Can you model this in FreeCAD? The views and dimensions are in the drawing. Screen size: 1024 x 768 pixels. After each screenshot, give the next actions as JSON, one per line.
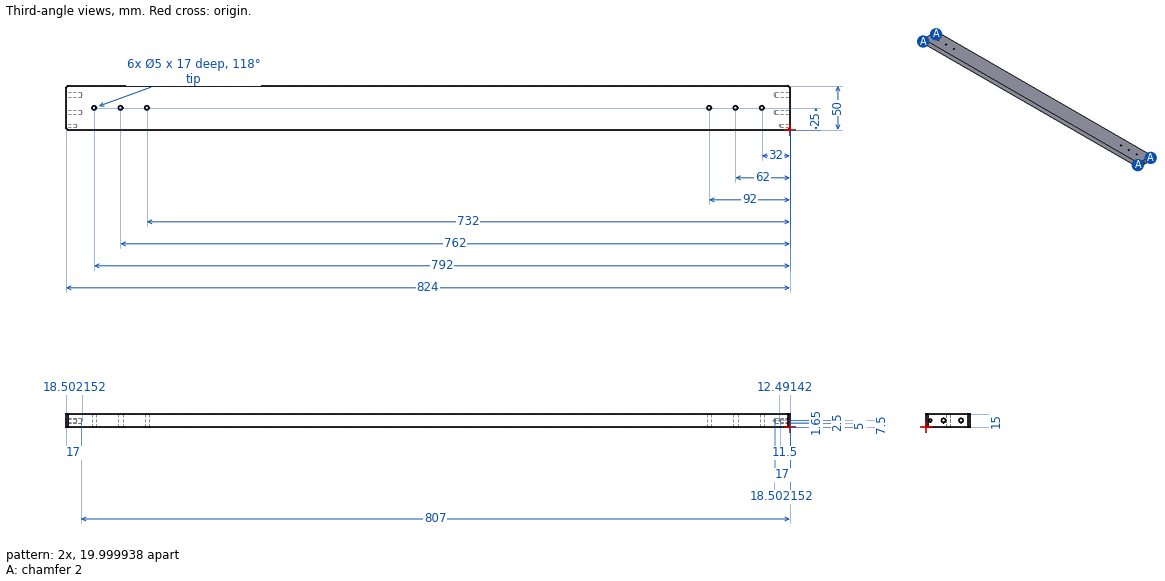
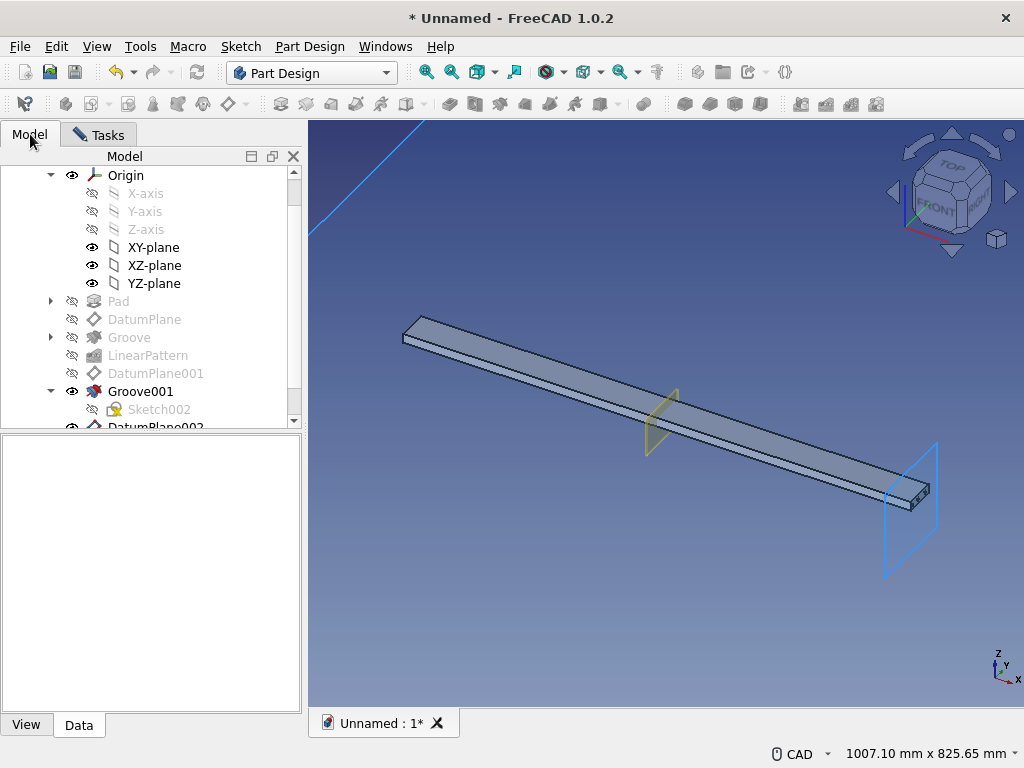
{"action": "left_click", "coordinate": [117, 427]}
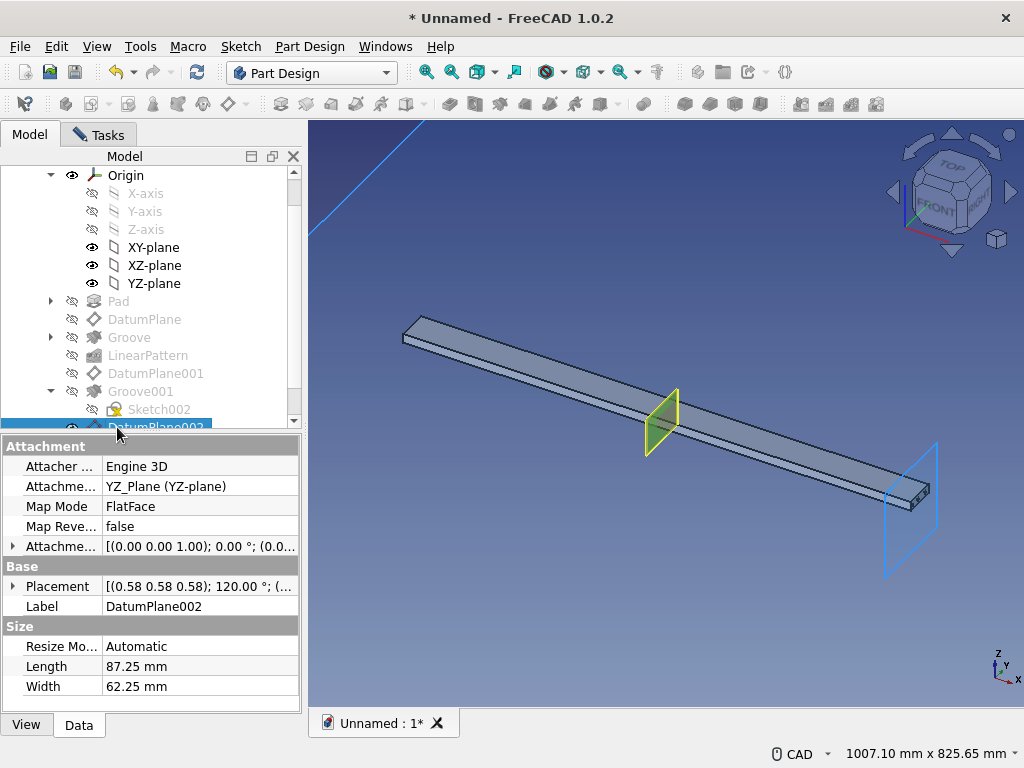
{"action": "left_click", "coordinate": [98, 134]}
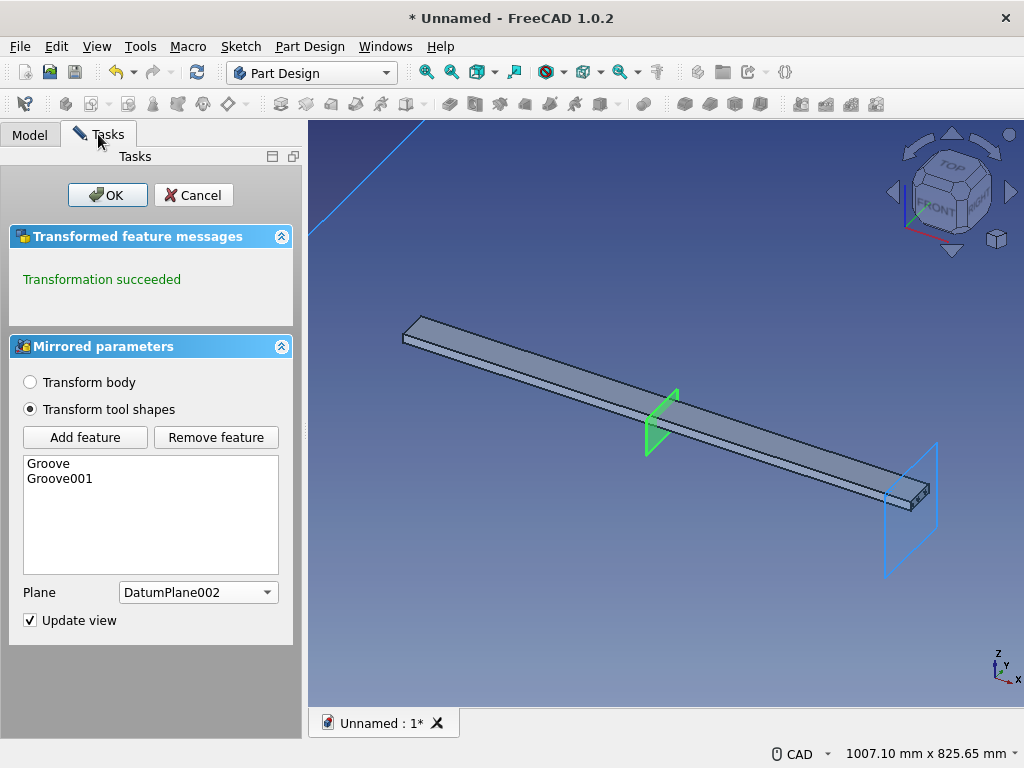
{"action": "left_click", "coordinate": [108, 195]}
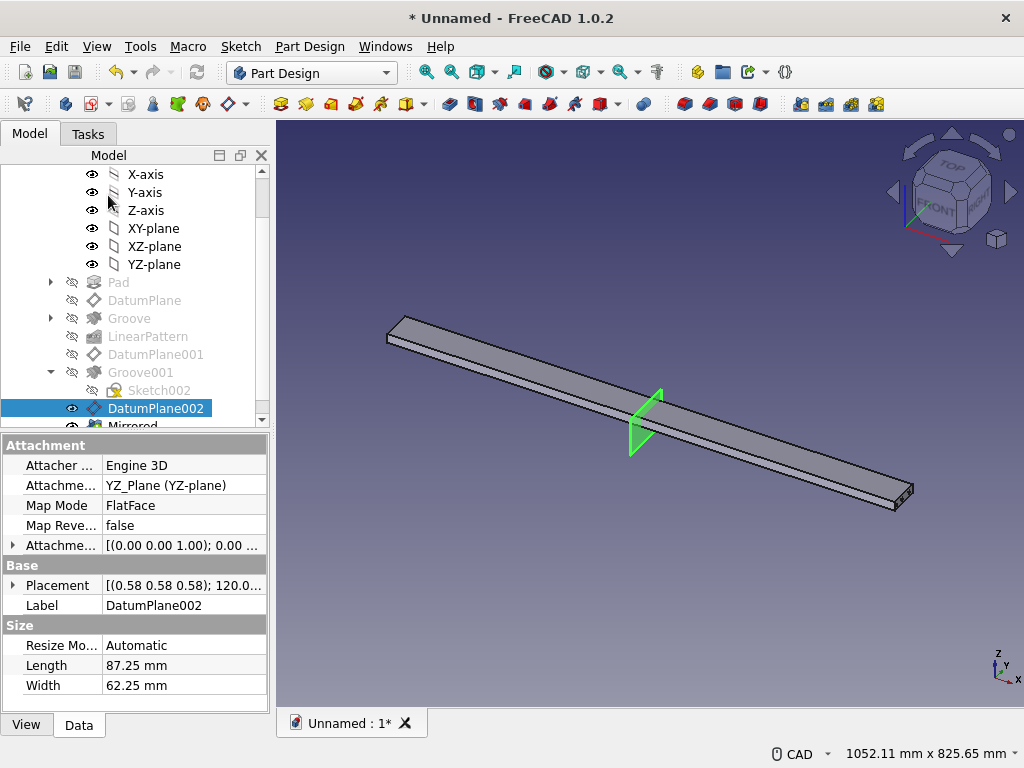
{"action": "left_click", "coordinate": [117, 408]}
{"action": "key", "text": "space"}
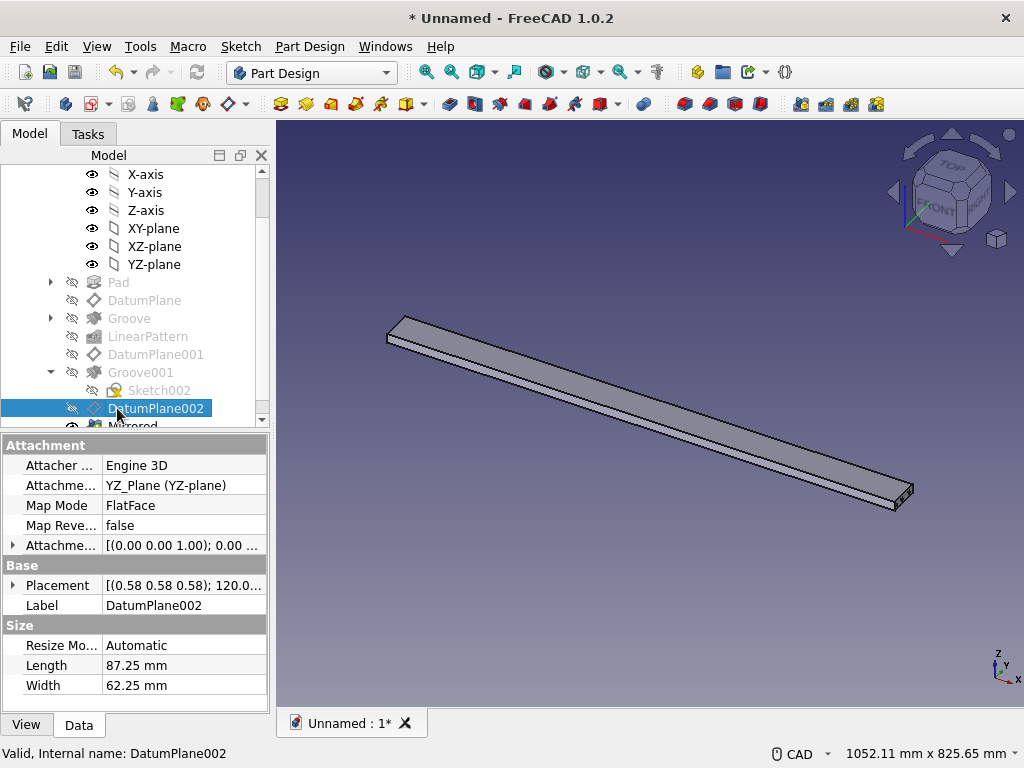
{"action": "scroll", "coordinate": [161, 296], "scroll_direction": "down", "scroll_amount": 3}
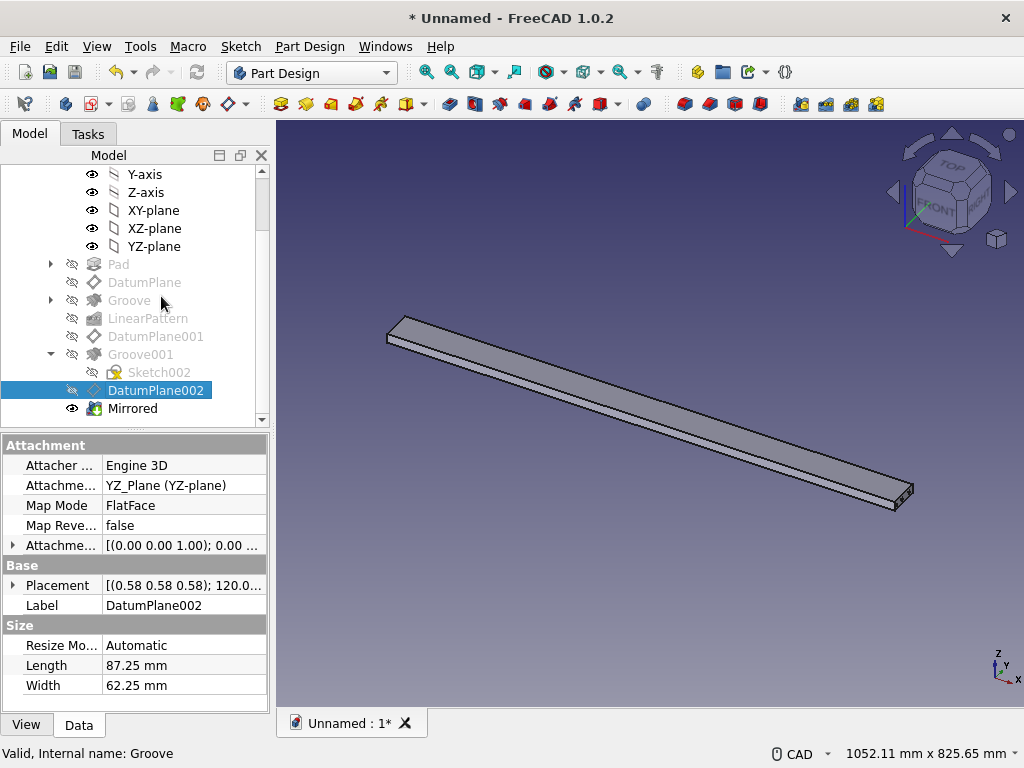
{"action": "scroll", "coordinate": [161, 296], "scroll_direction": "up", "scroll_amount": 15}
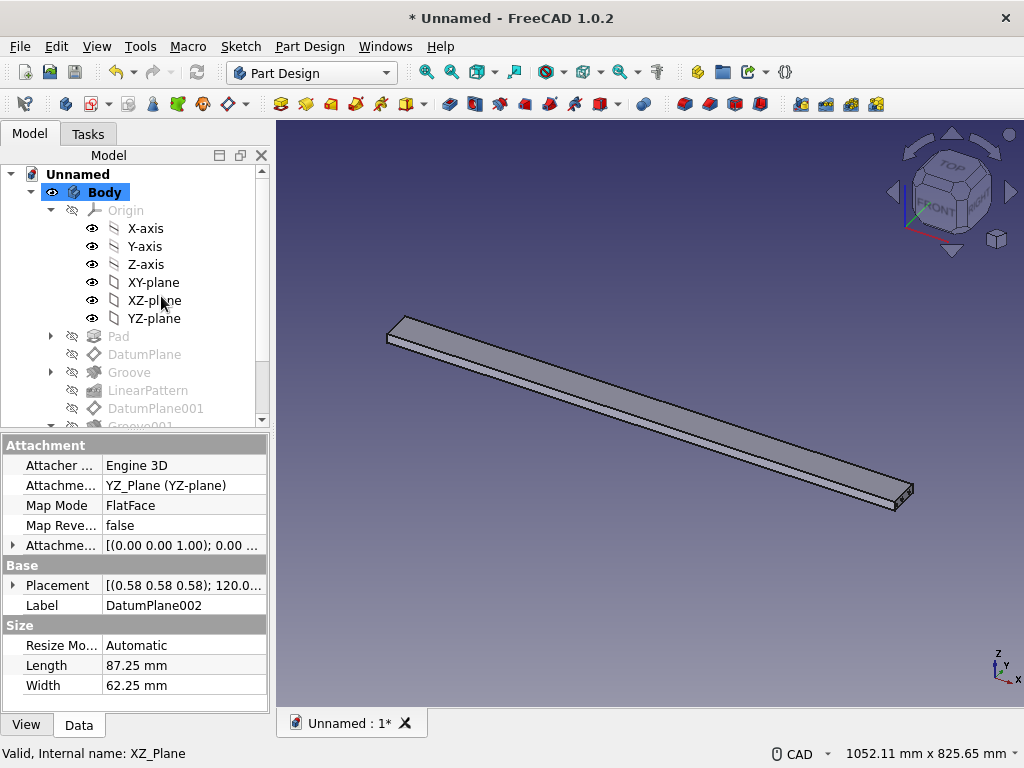
{"action": "left_click", "coordinate": [137, 300]}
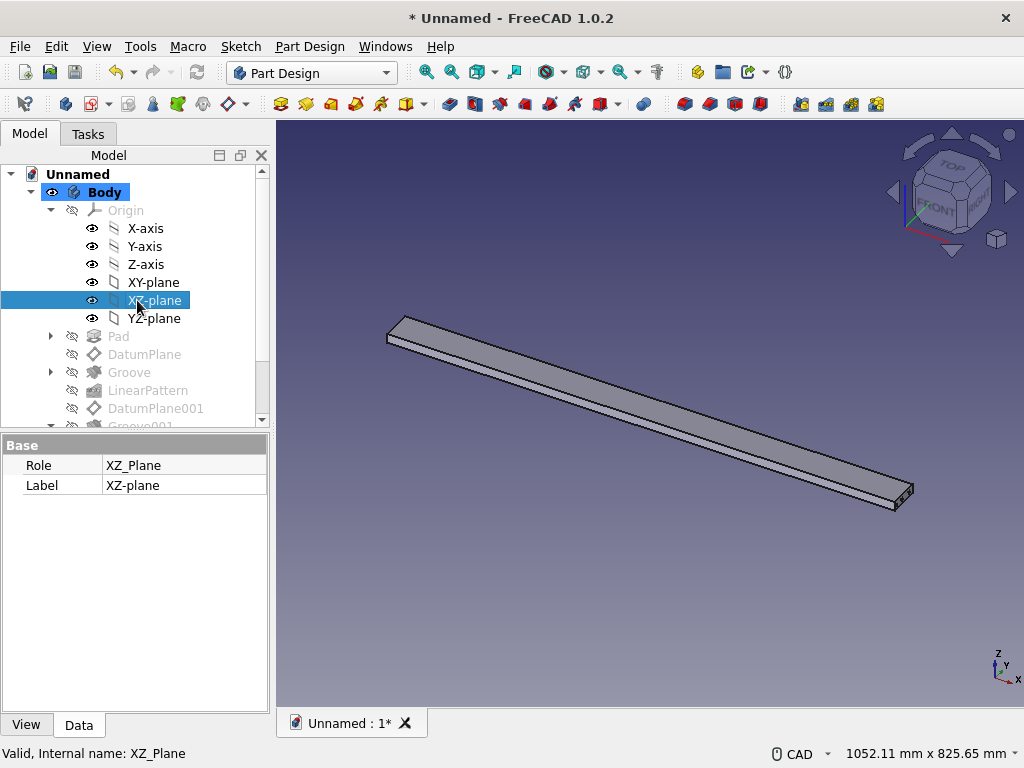
{"action": "left_click", "coordinate": [228, 104]}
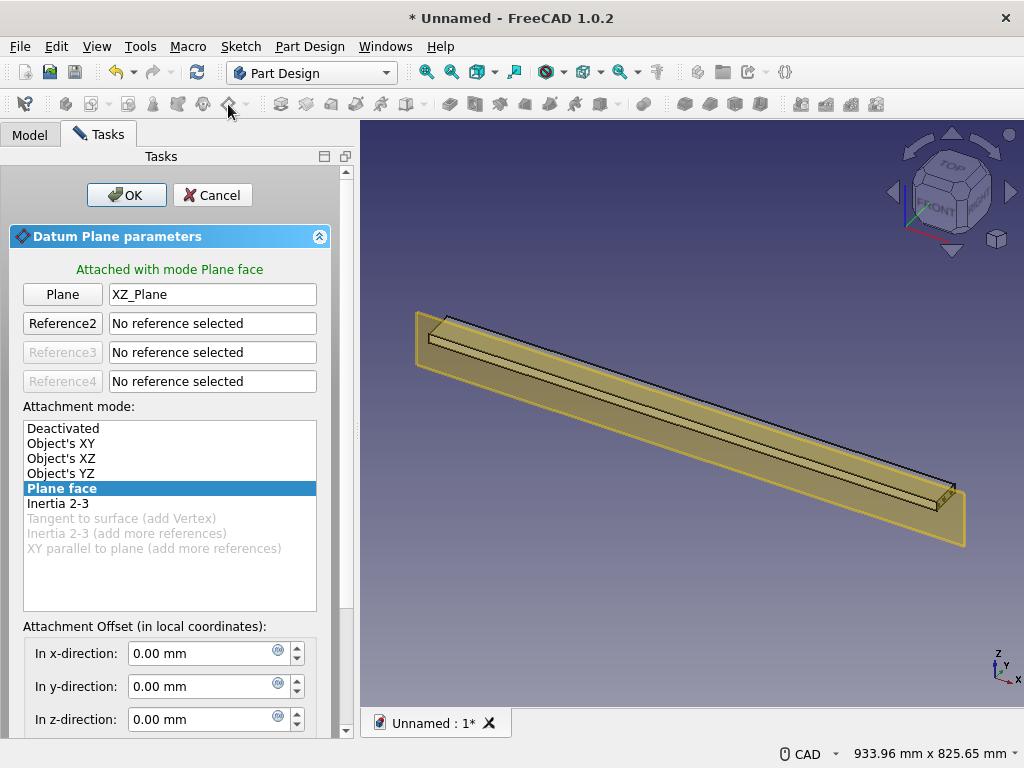
{"action": "triple_click", "coordinate": [210, 720]}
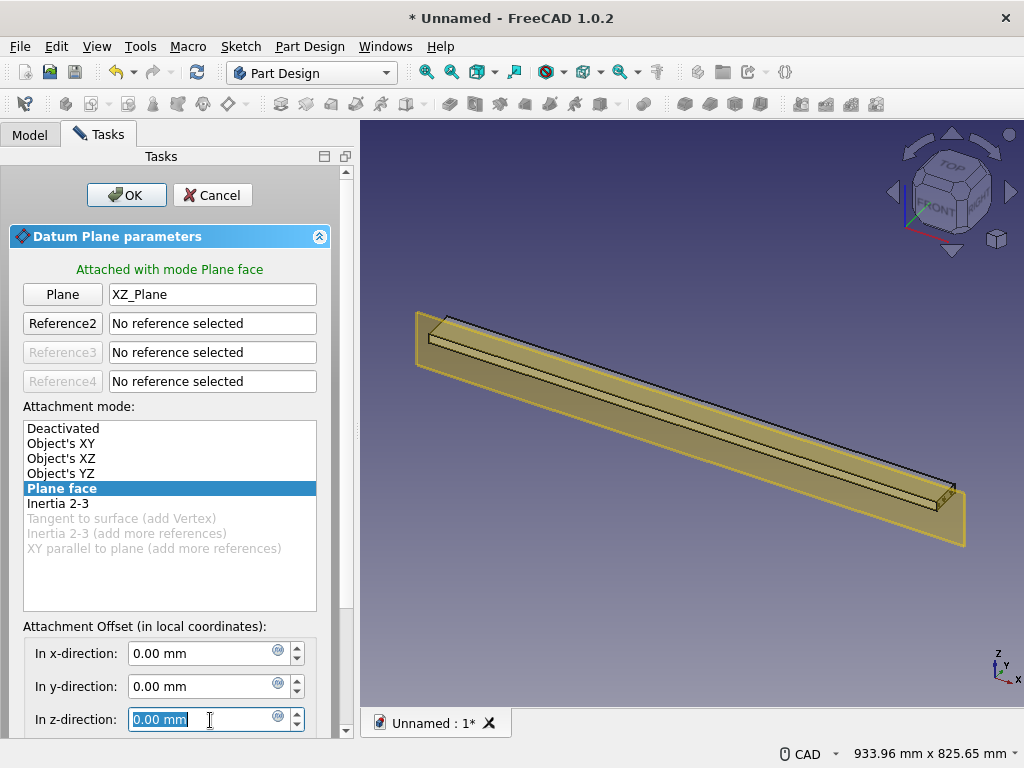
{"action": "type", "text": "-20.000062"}
{"action": "key", "text": "Tab"}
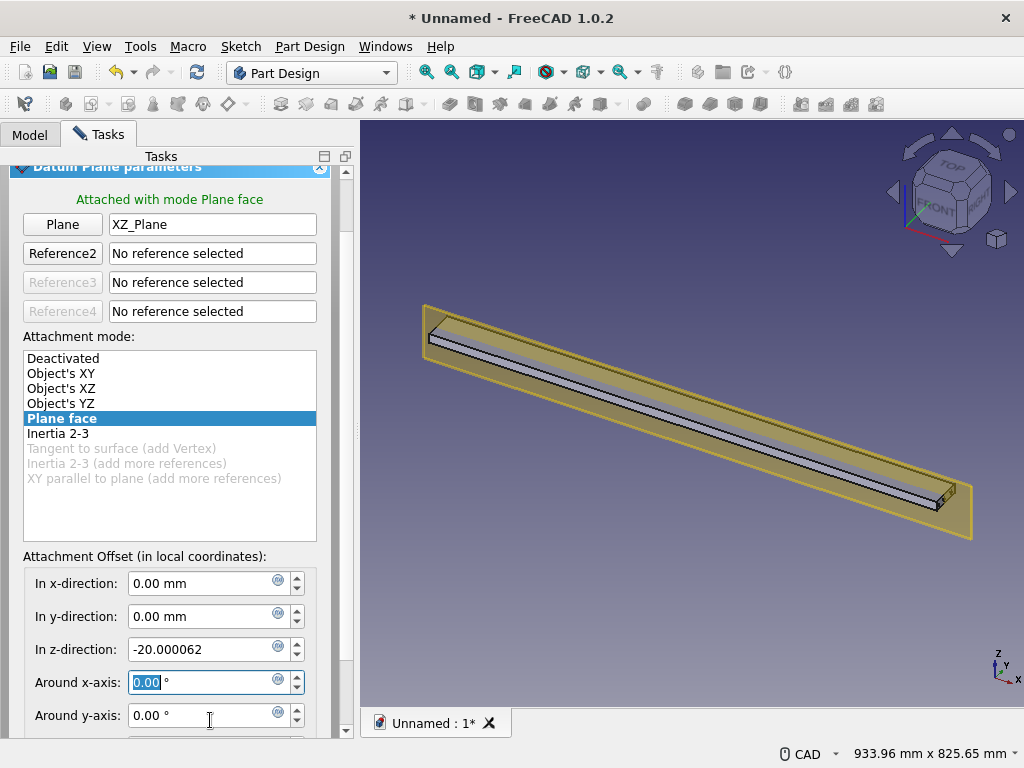
{"action": "scroll", "coordinate": [346, 452], "scroll_direction": "up", "scroll_amount": 2}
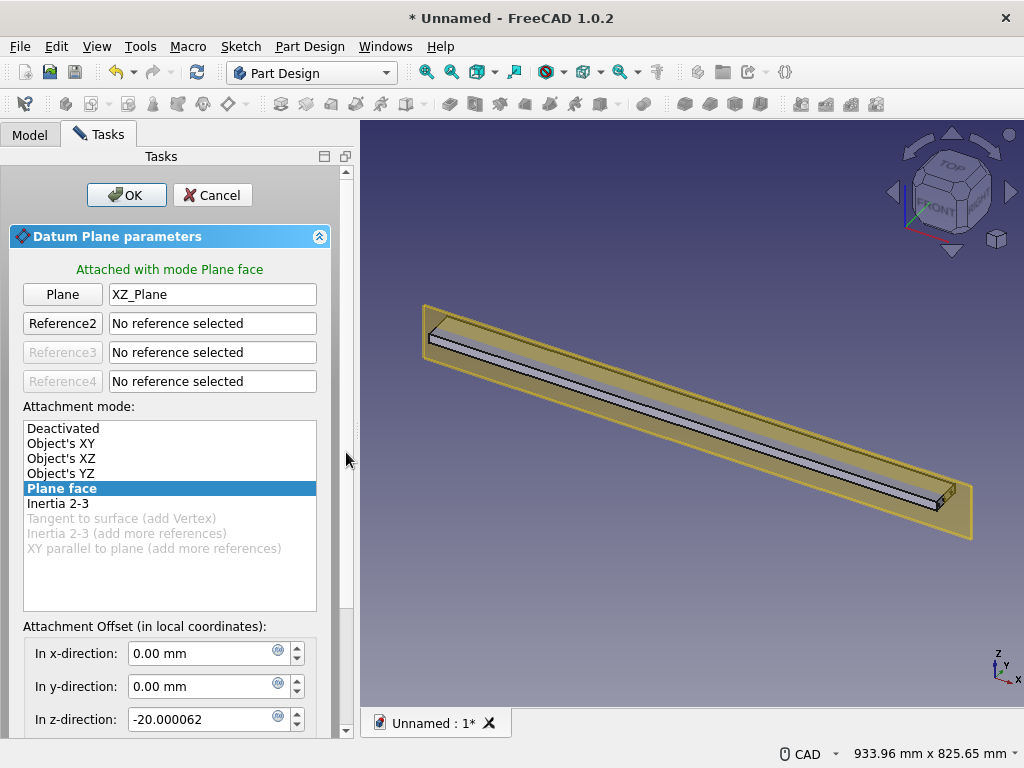
{"action": "left_click", "coordinate": [127, 195]}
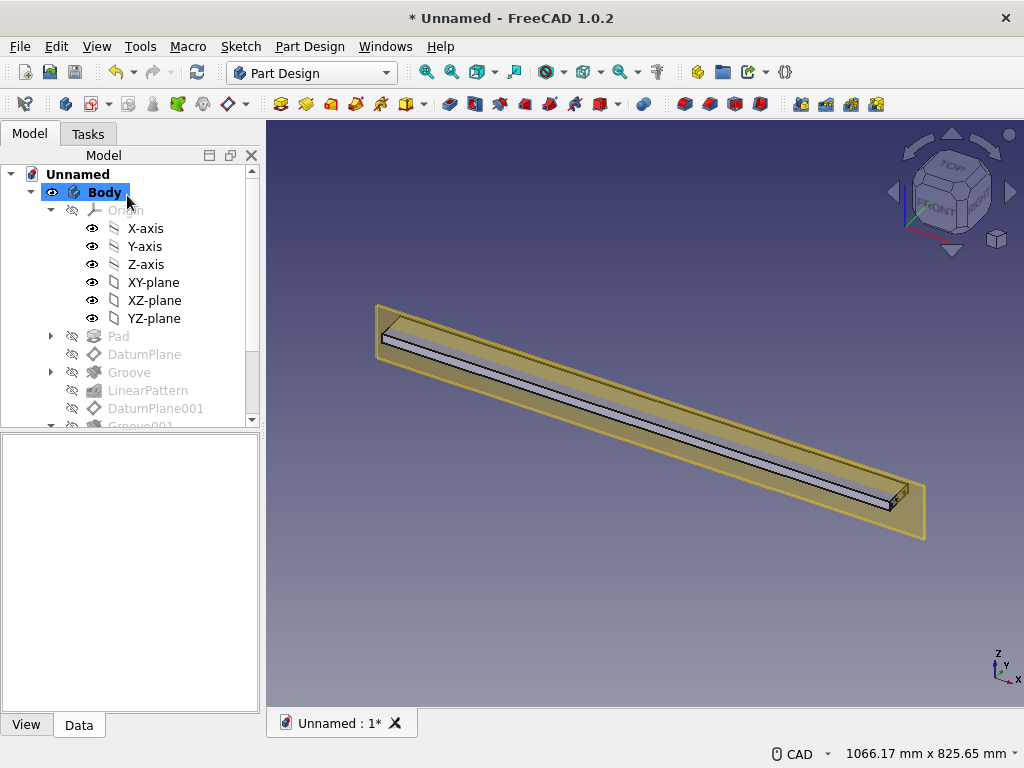
{"action": "scroll", "coordinate": [101, 296], "scroll_direction": "down", "scroll_amount": 3}